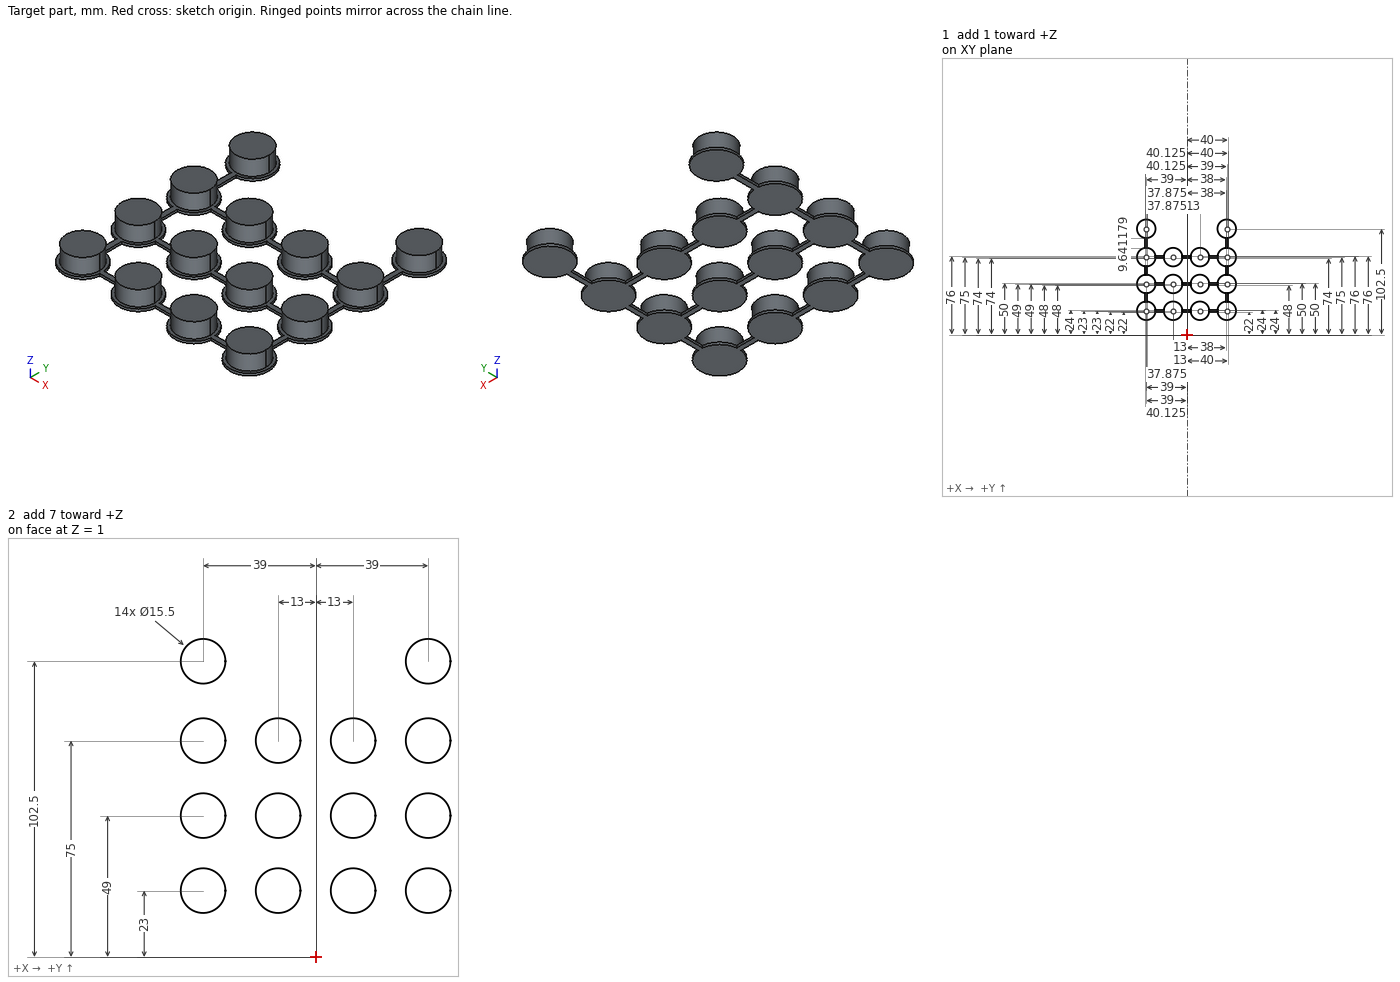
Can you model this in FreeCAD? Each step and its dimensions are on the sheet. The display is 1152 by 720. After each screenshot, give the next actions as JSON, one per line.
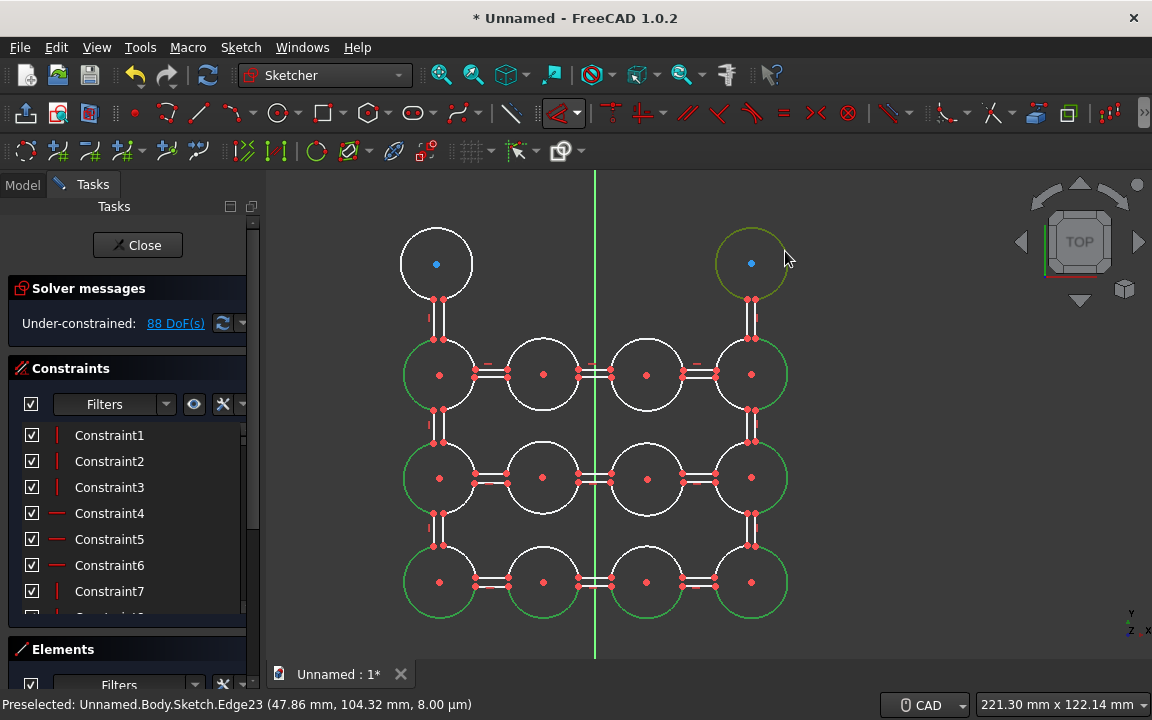
{"action": "left_click", "coordinate": [734, 343]}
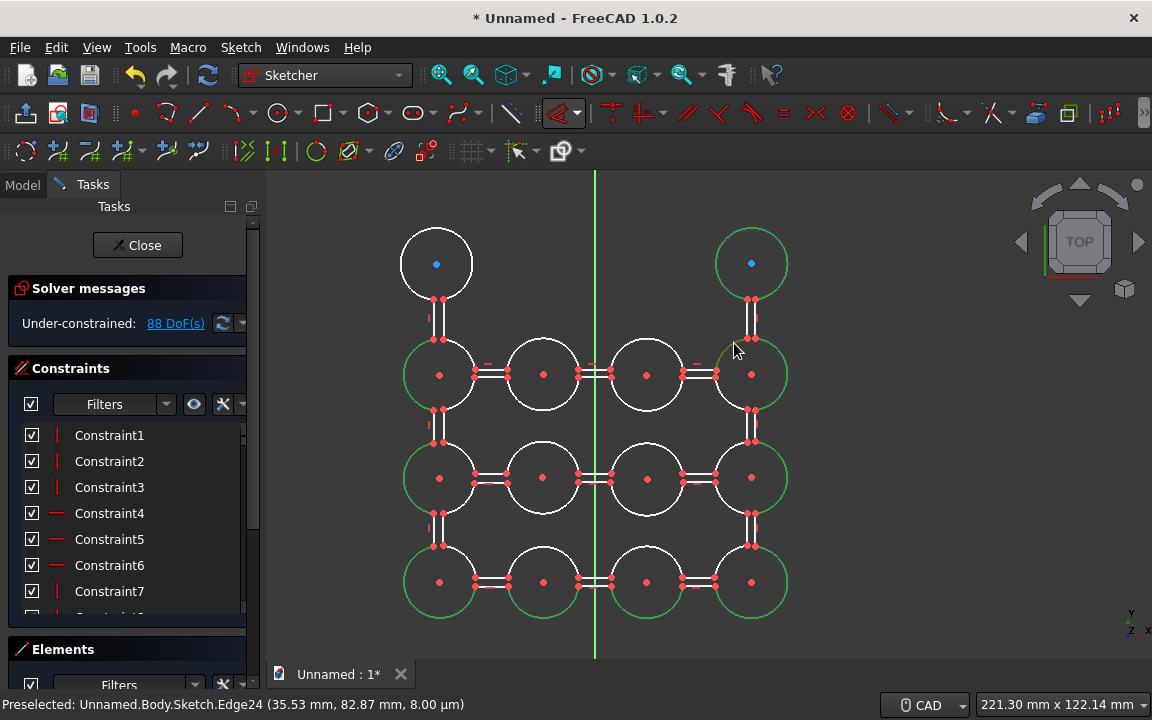
{"action": "left_click", "coordinate": [667, 344]}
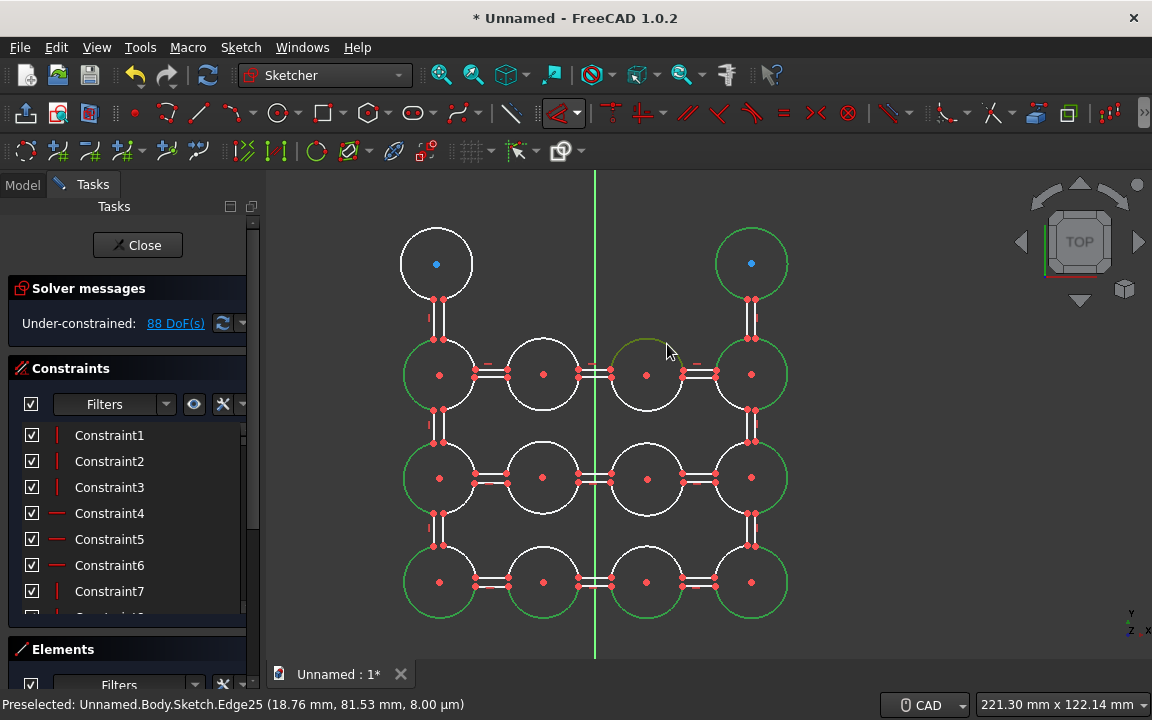
{"action": "left_click", "coordinate": [563, 344]}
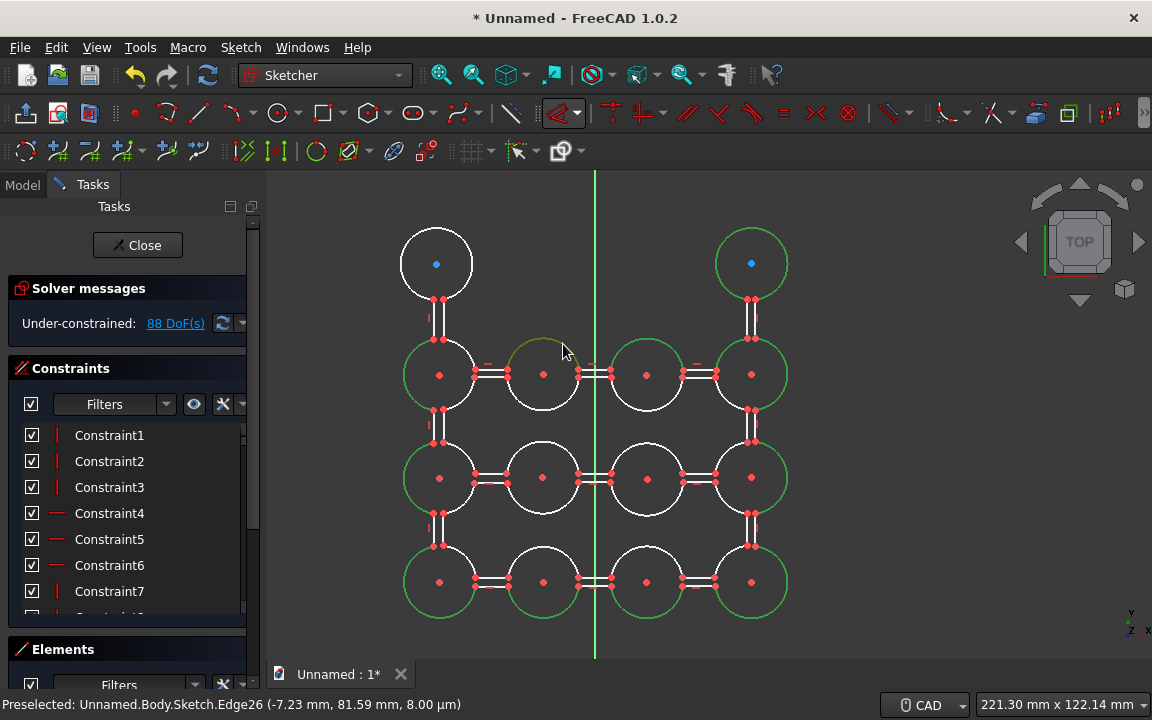
{"action": "left_click", "coordinate": [470, 357]}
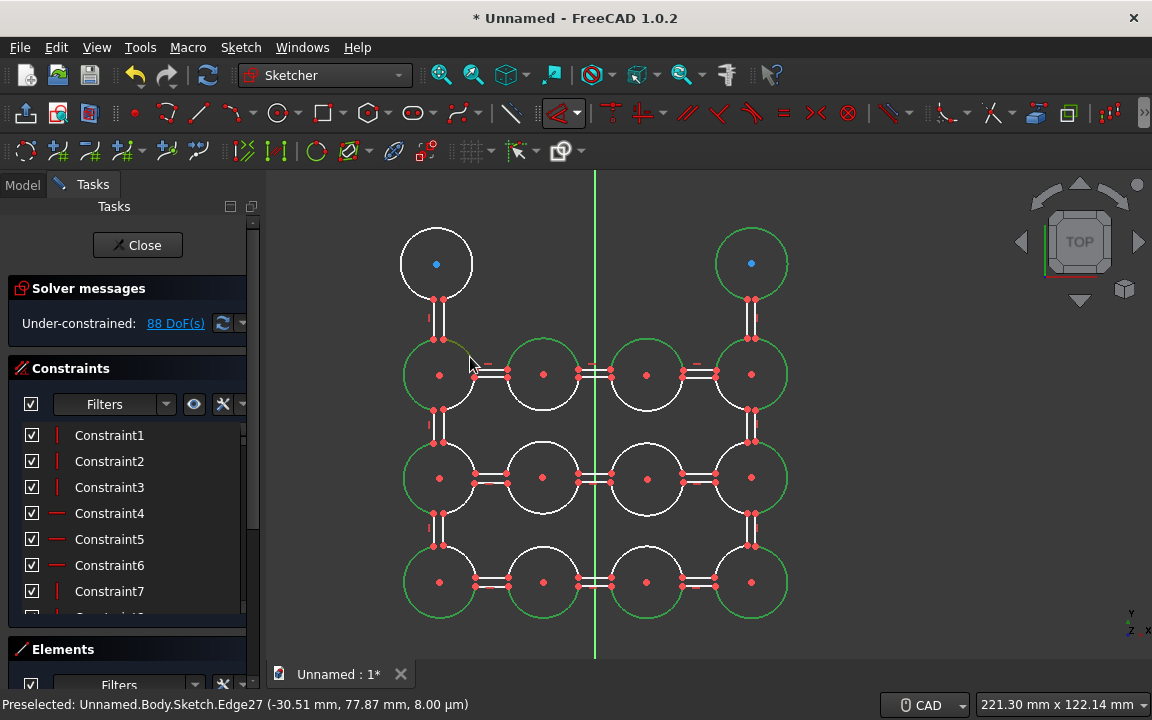
{"action": "left_click", "coordinate": [469, 249]}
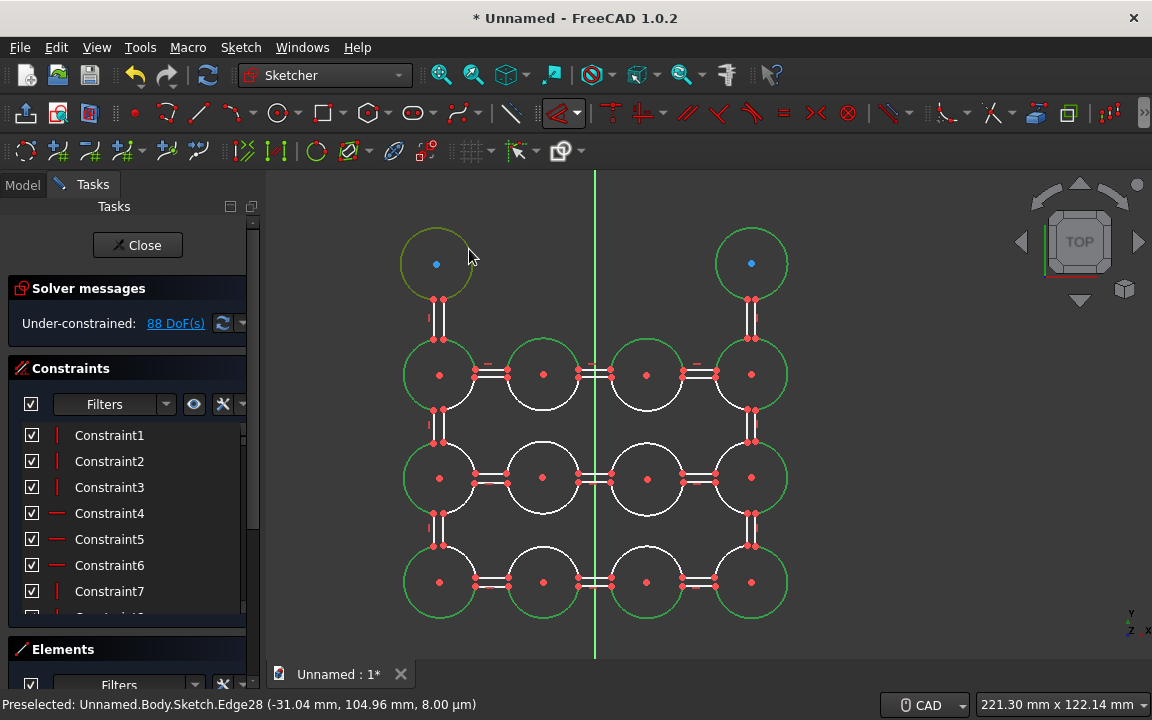
{"action": "left_click", "coordinate": [524, 508]}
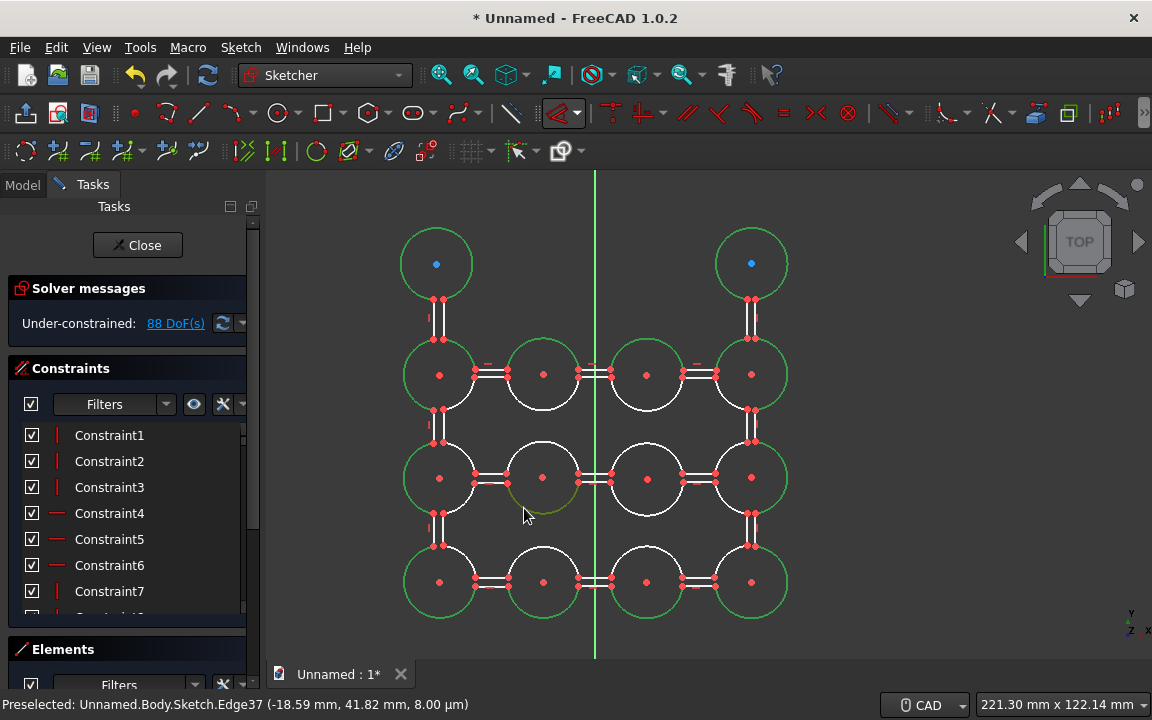
{"action": "left_click", "coordinate": [627, 509]}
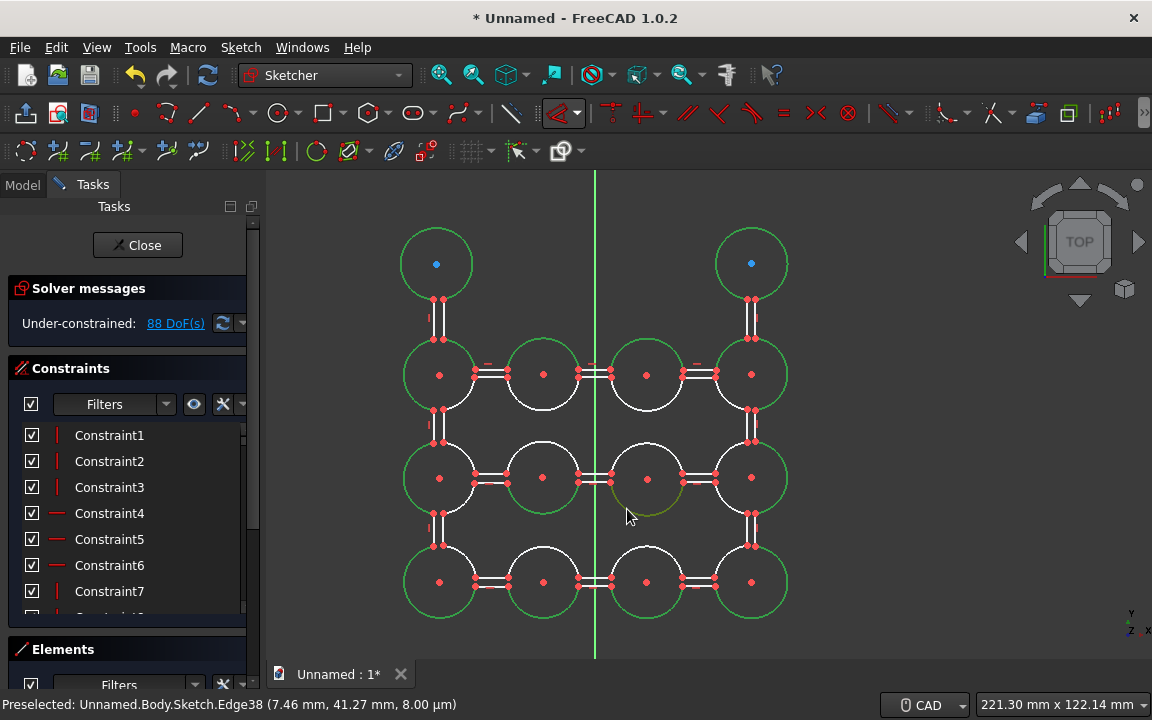
{"action": "left_click", "coordinate": [720, 496]}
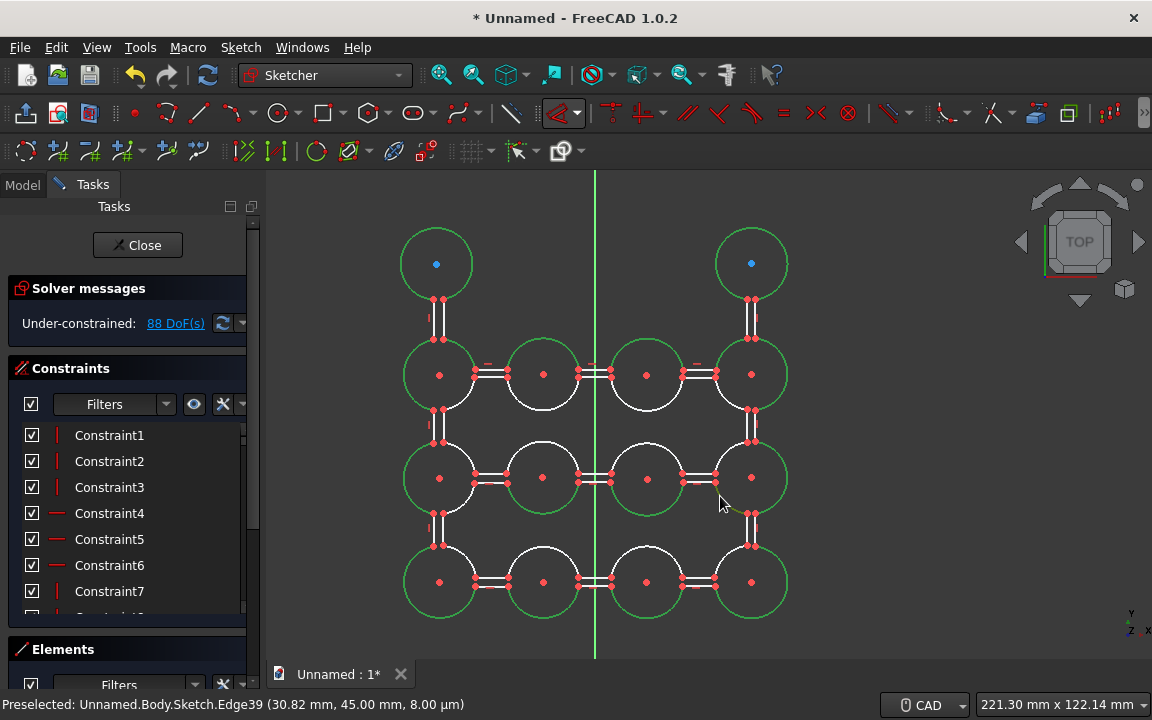
{"action": "left_click", "coordinate": [733, 550]}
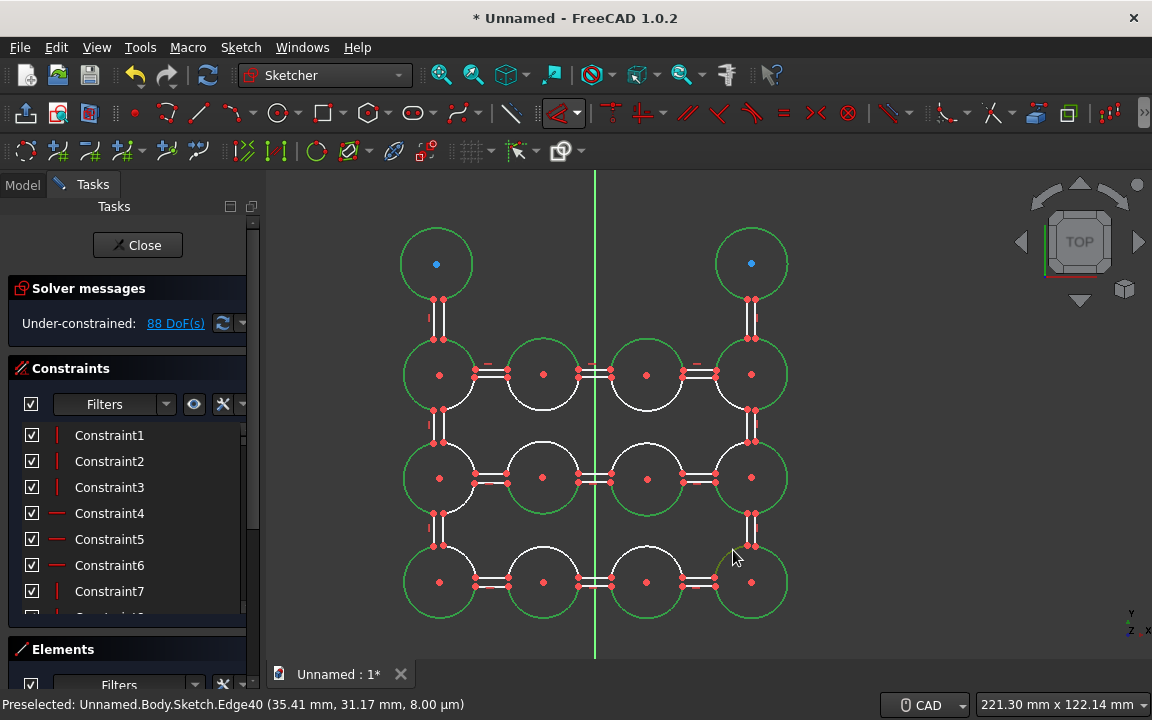
{"action": "left_click", "coordinate": [666, 552]}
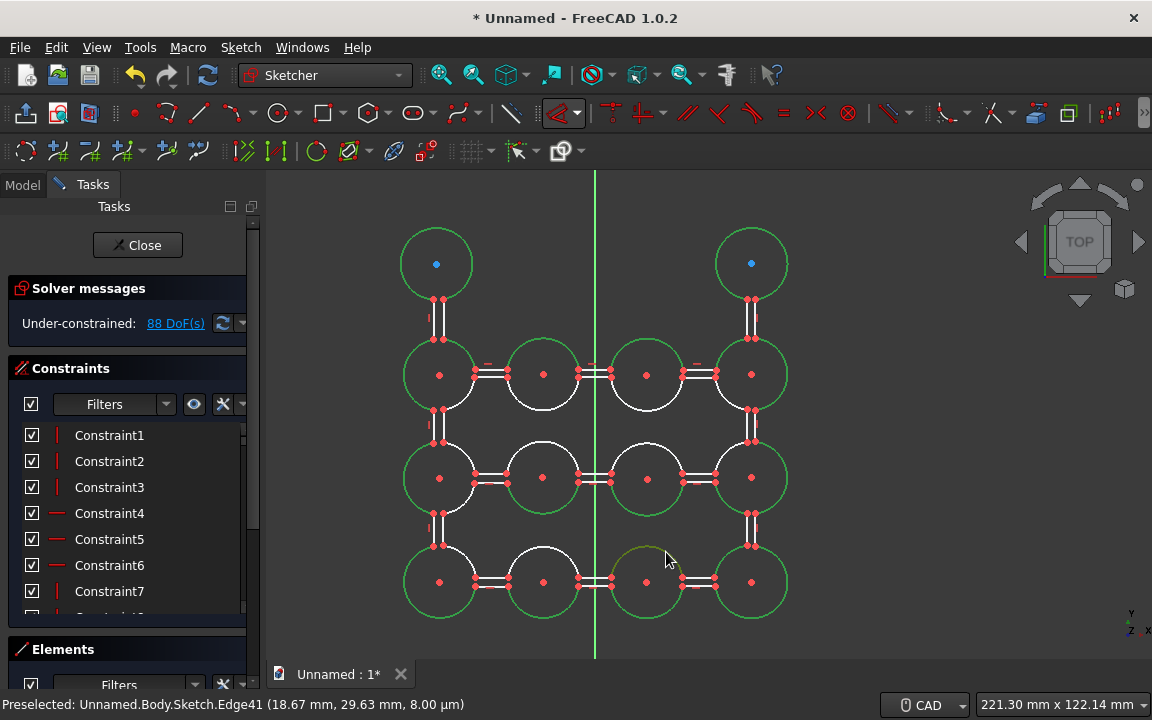
{"action": "left_click", "coordinate": [563, 553]}